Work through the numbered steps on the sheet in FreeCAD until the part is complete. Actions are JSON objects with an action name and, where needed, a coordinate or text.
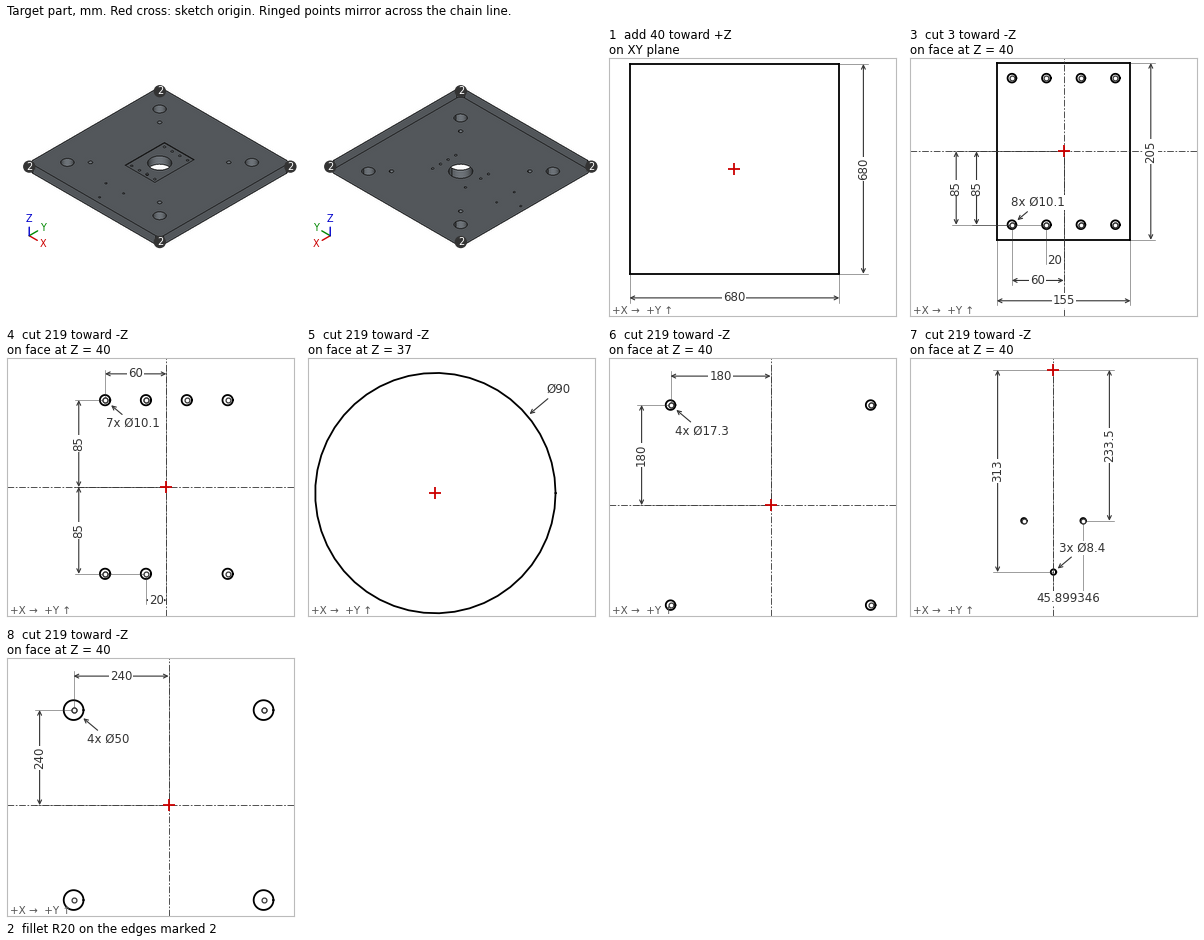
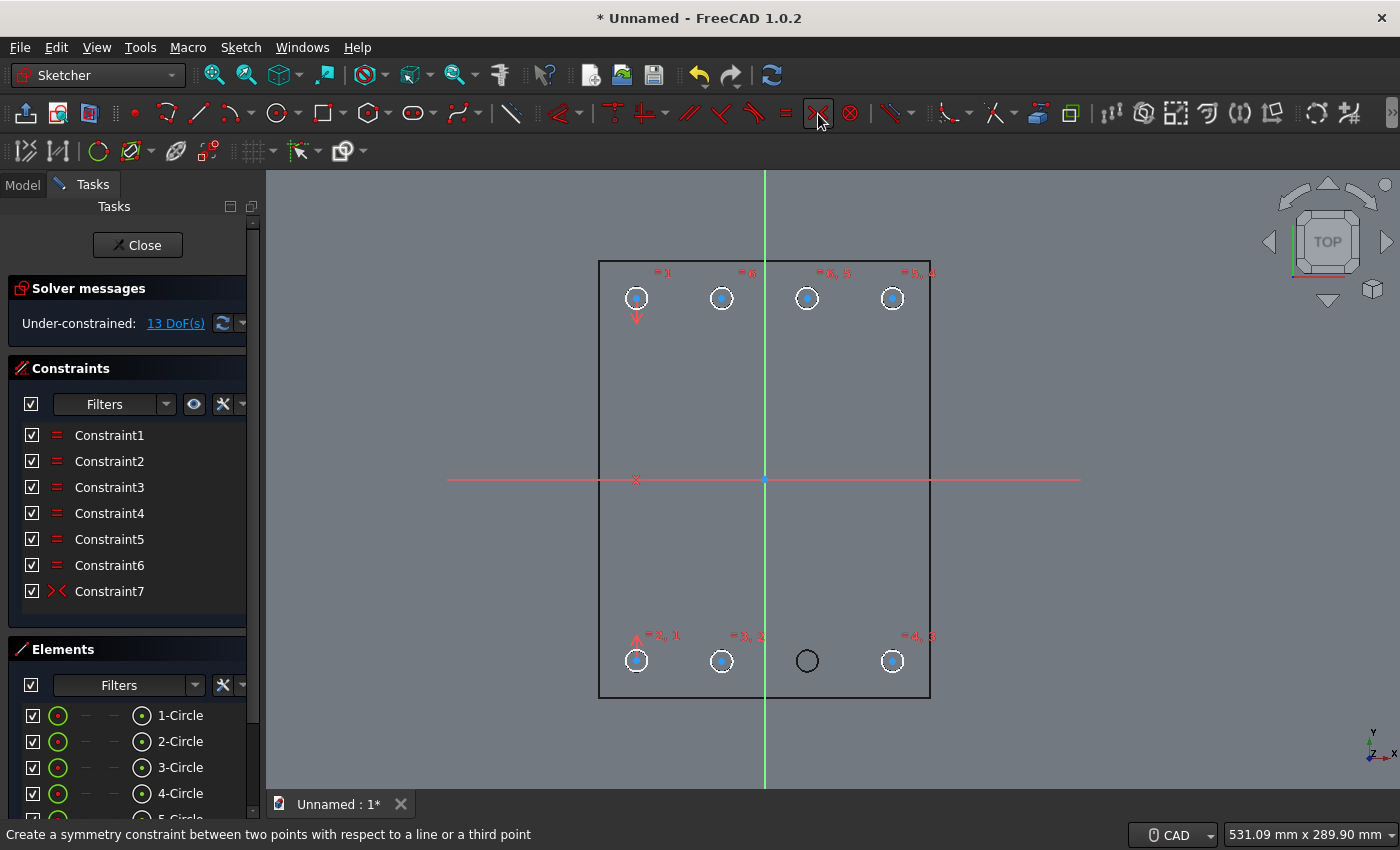
{"action": "left_click", "coordinate": [637, 661]}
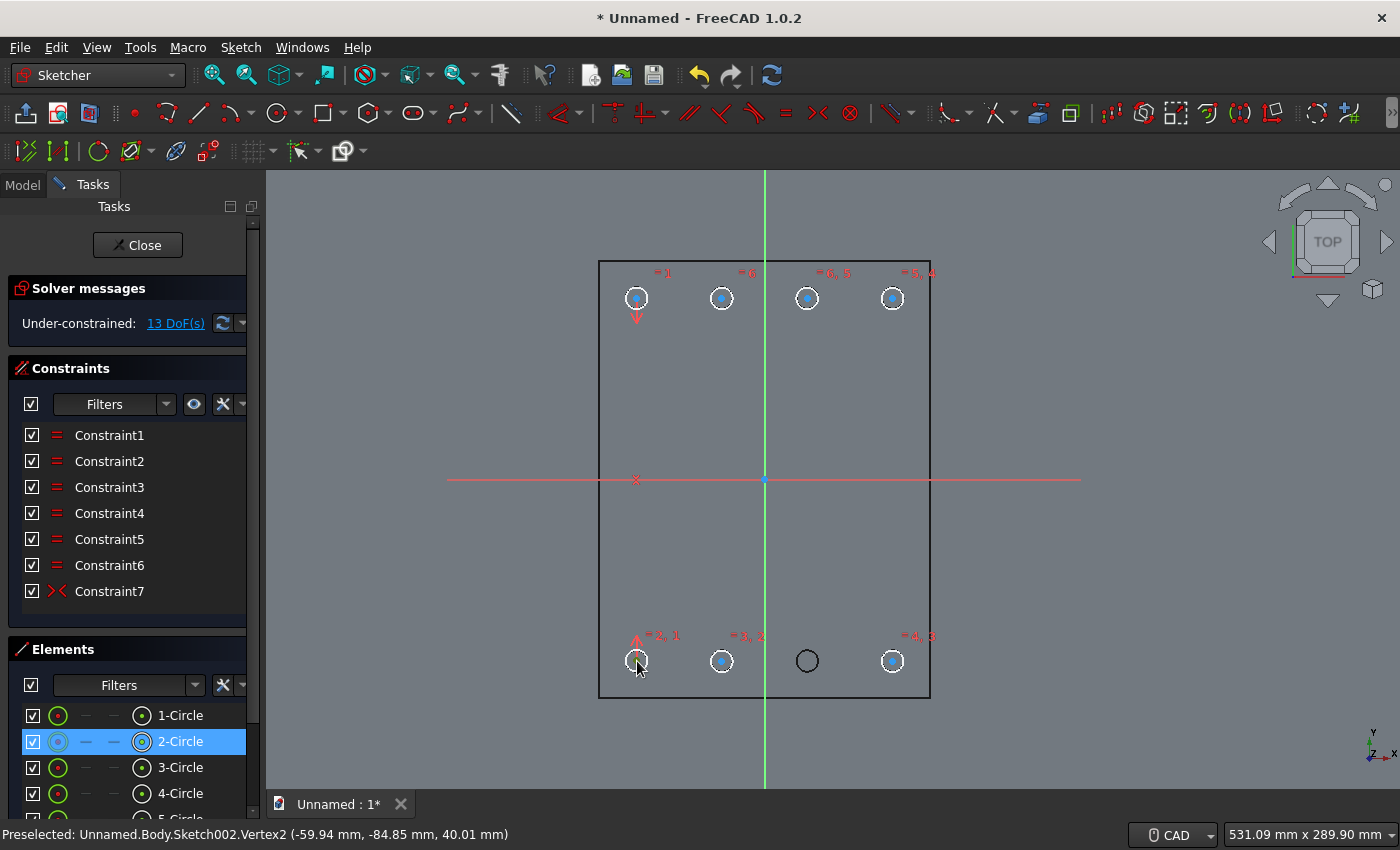
{"action": "left_click", "coordinate": [893, 661]}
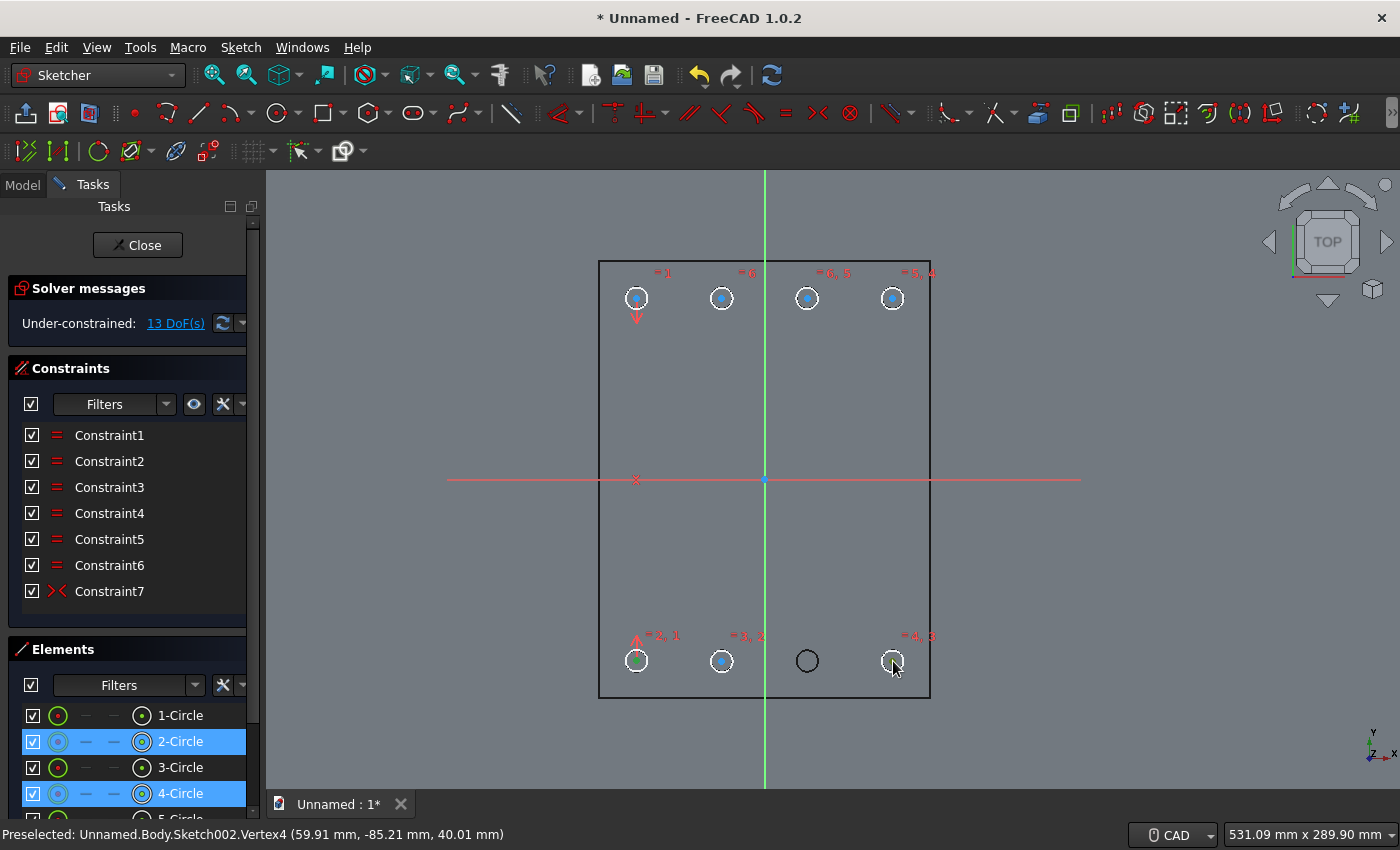
{"action": "left_click", "coordinate": [765, 721]}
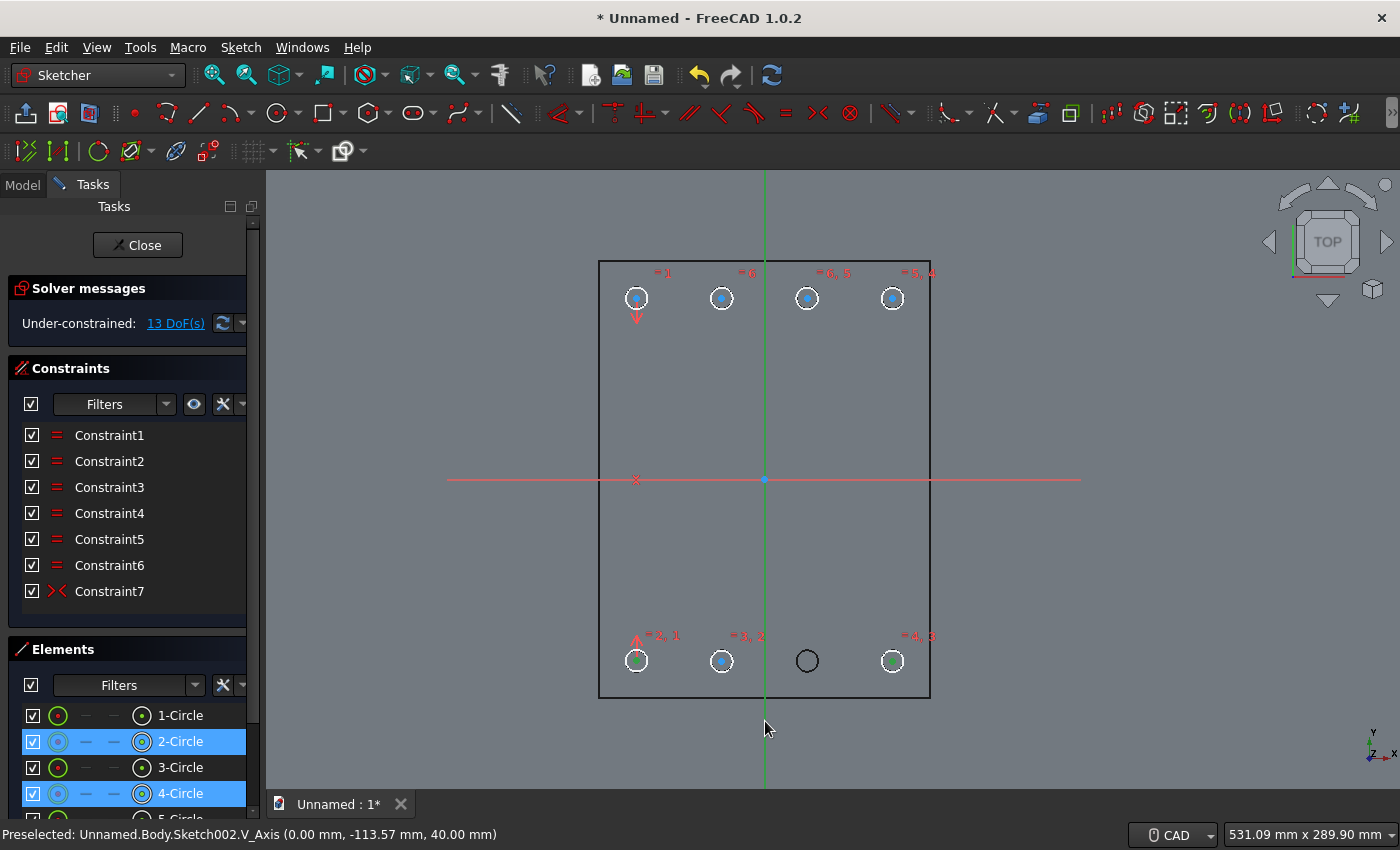
{"action": "left_click", "coordinate": [818, 114]}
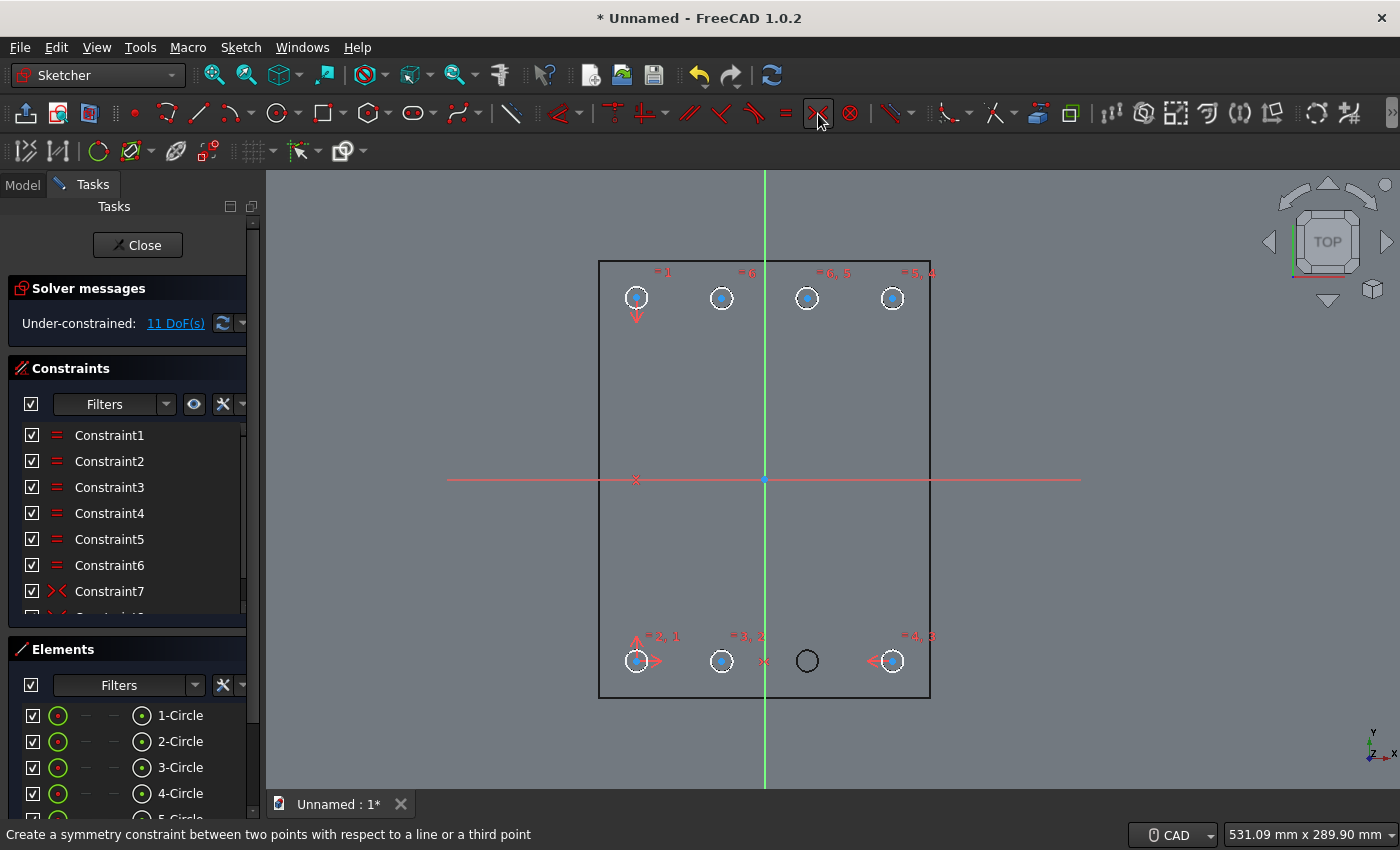
{"action": "left_click", "coordinate": [637, 298]}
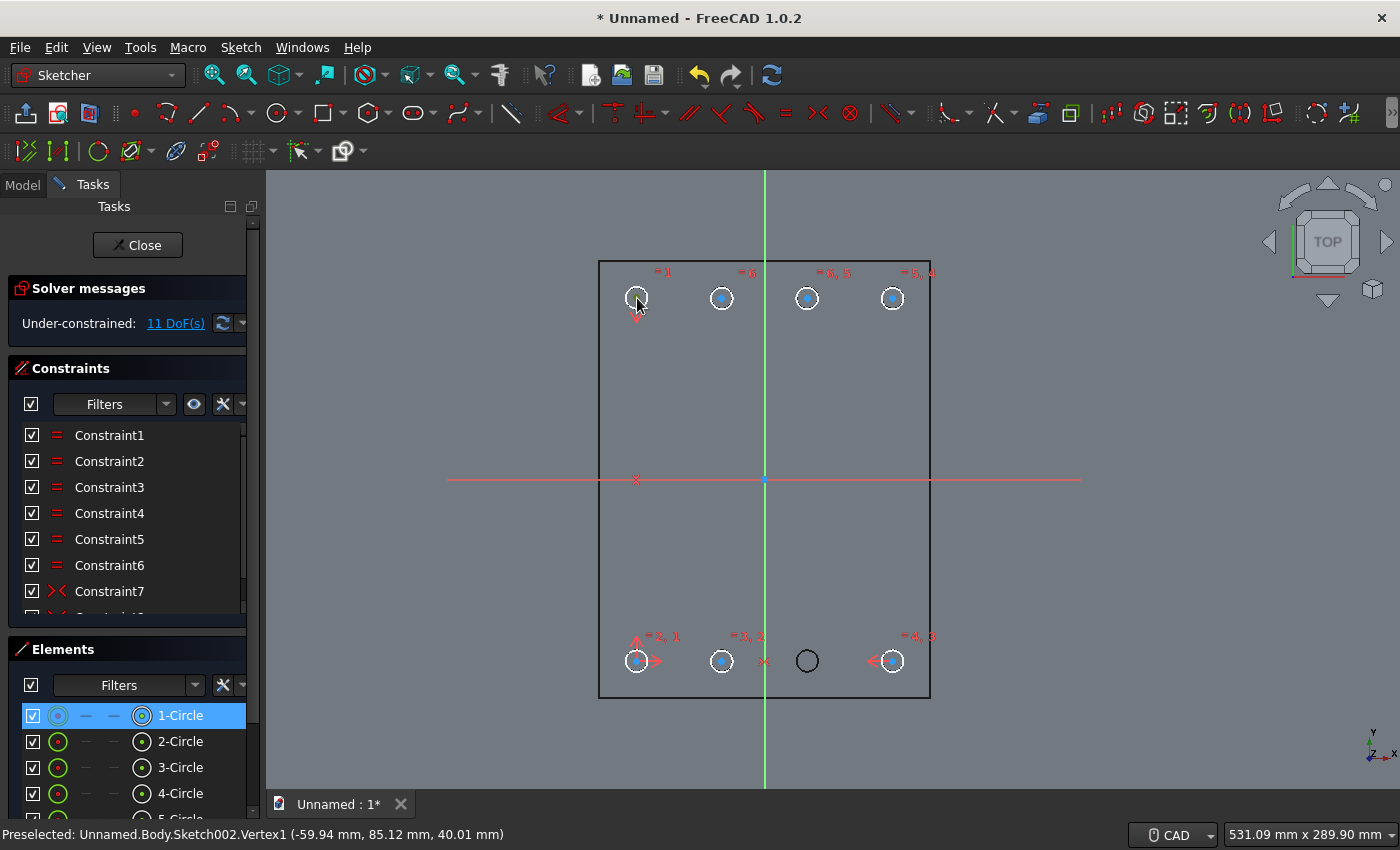
{"action": "left_click", "coordinate": [893, 299]}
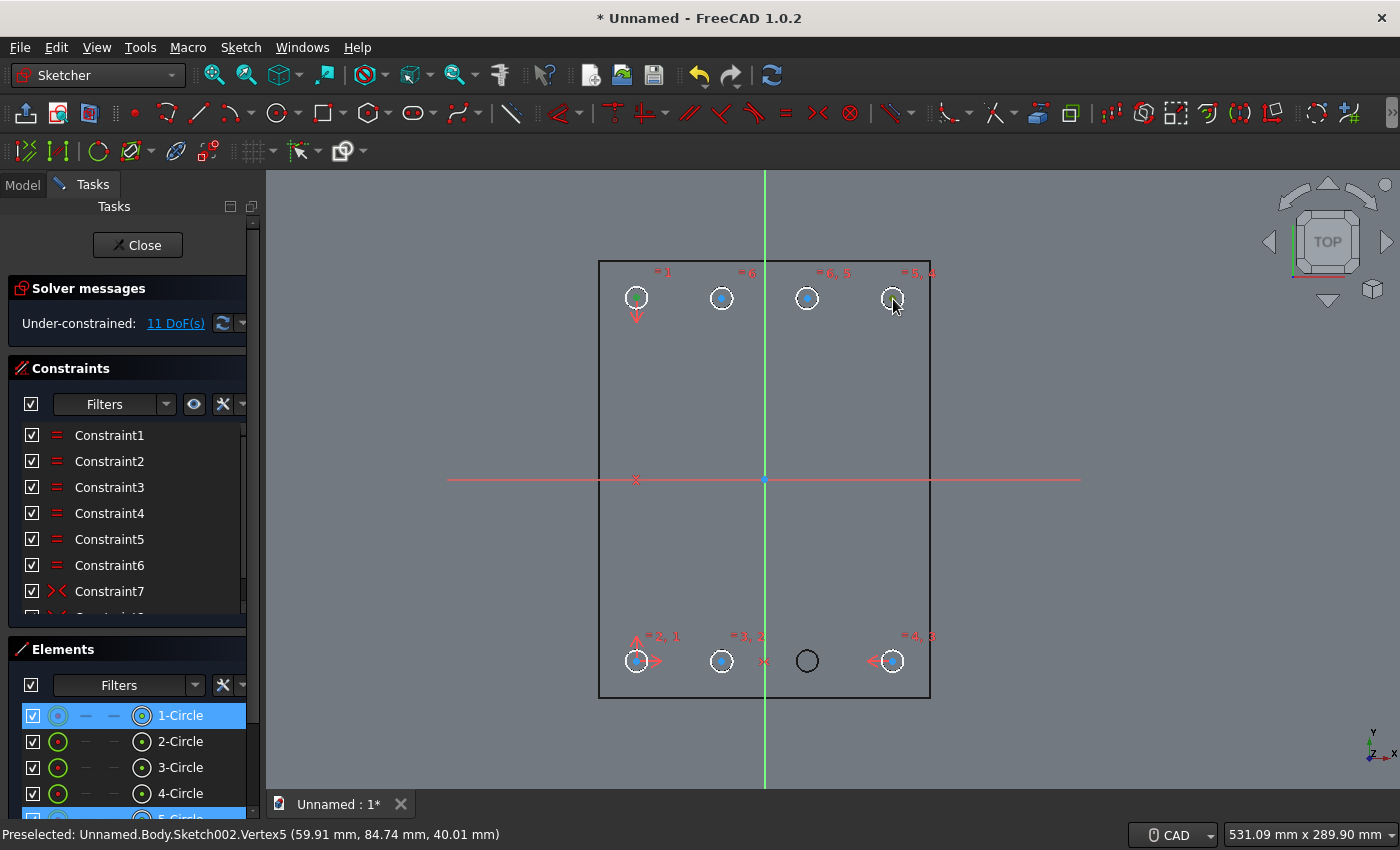
{"action": "left_click", "coordinate": [765, 721]}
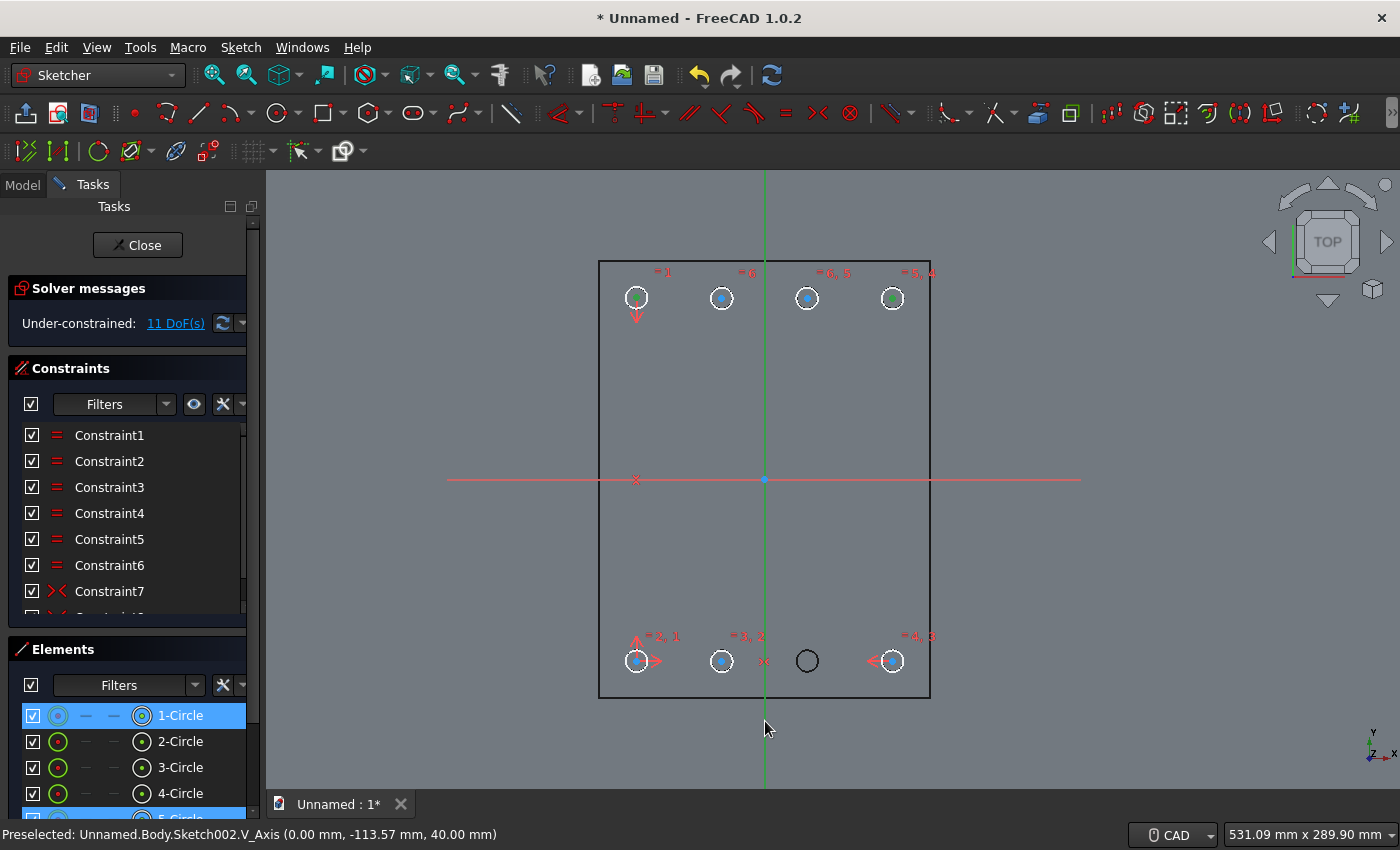
{"action": "left_click", "coordinate": [818, 114]}